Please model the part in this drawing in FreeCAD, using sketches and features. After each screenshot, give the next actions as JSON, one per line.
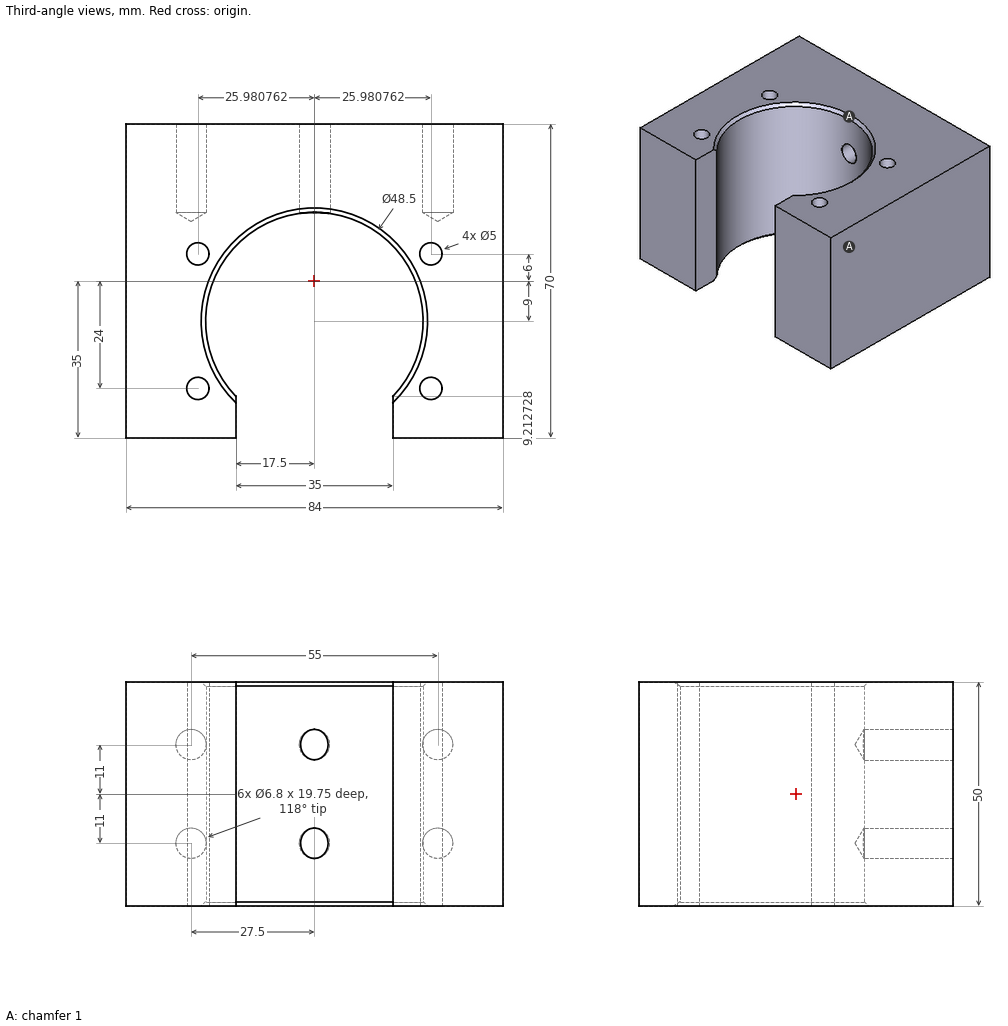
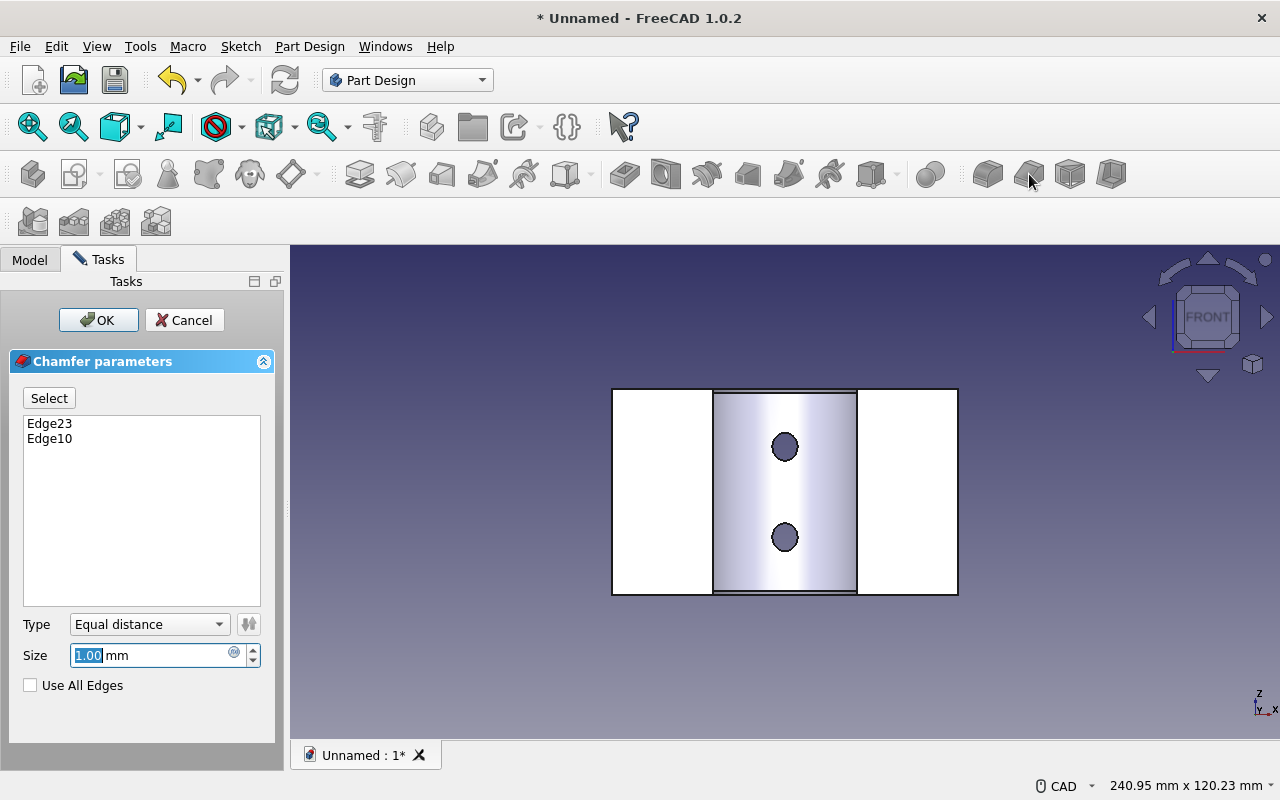
{"action": "type", "text": "1"}
{"action": "key", "text": "Tab"}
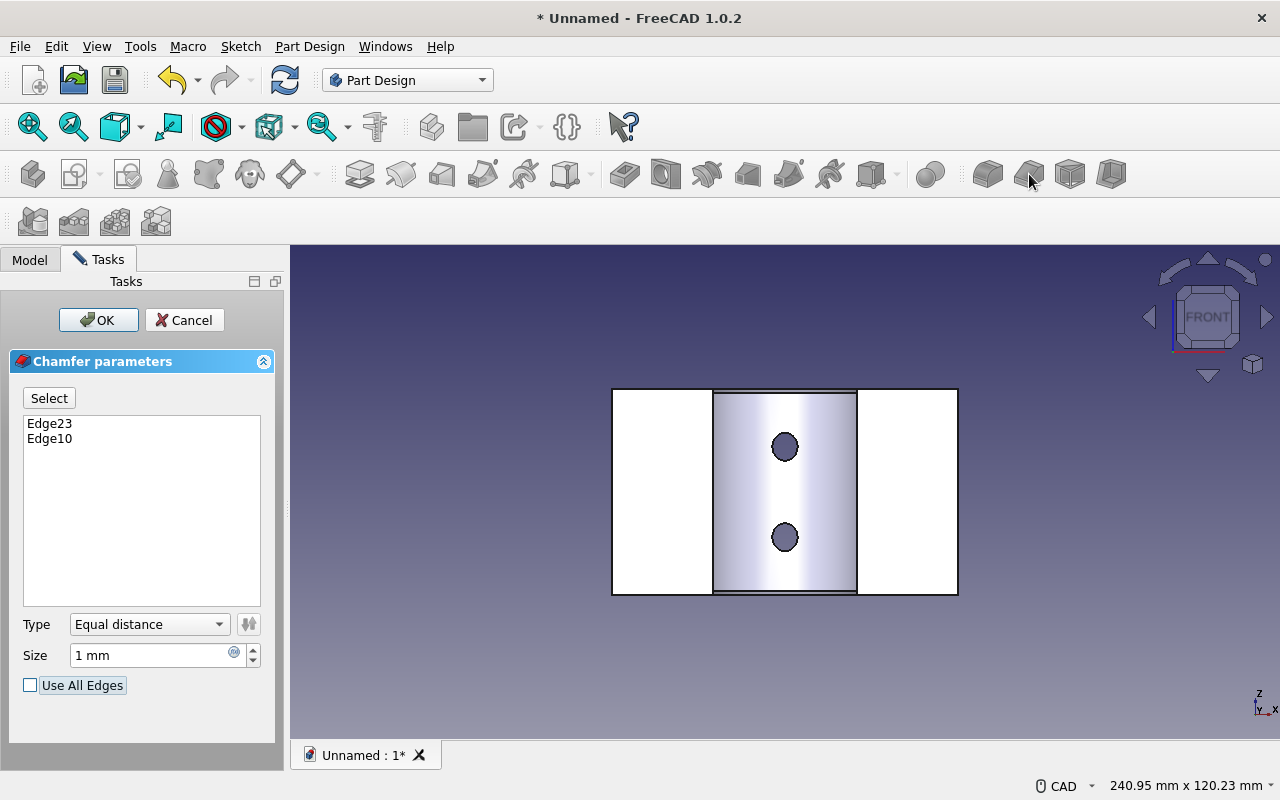
{"action": "left_click", "coordinate": [99, 320]}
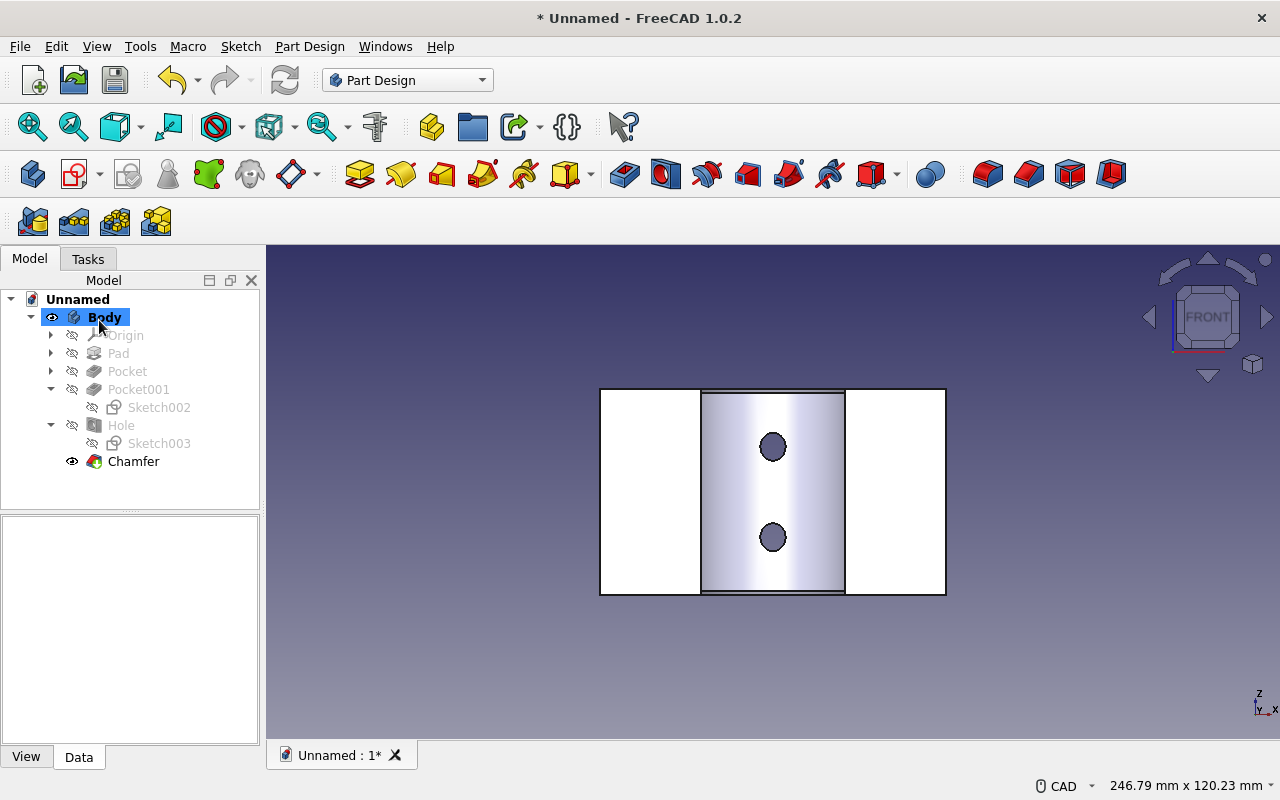
{"action": "key", "text": "0"}